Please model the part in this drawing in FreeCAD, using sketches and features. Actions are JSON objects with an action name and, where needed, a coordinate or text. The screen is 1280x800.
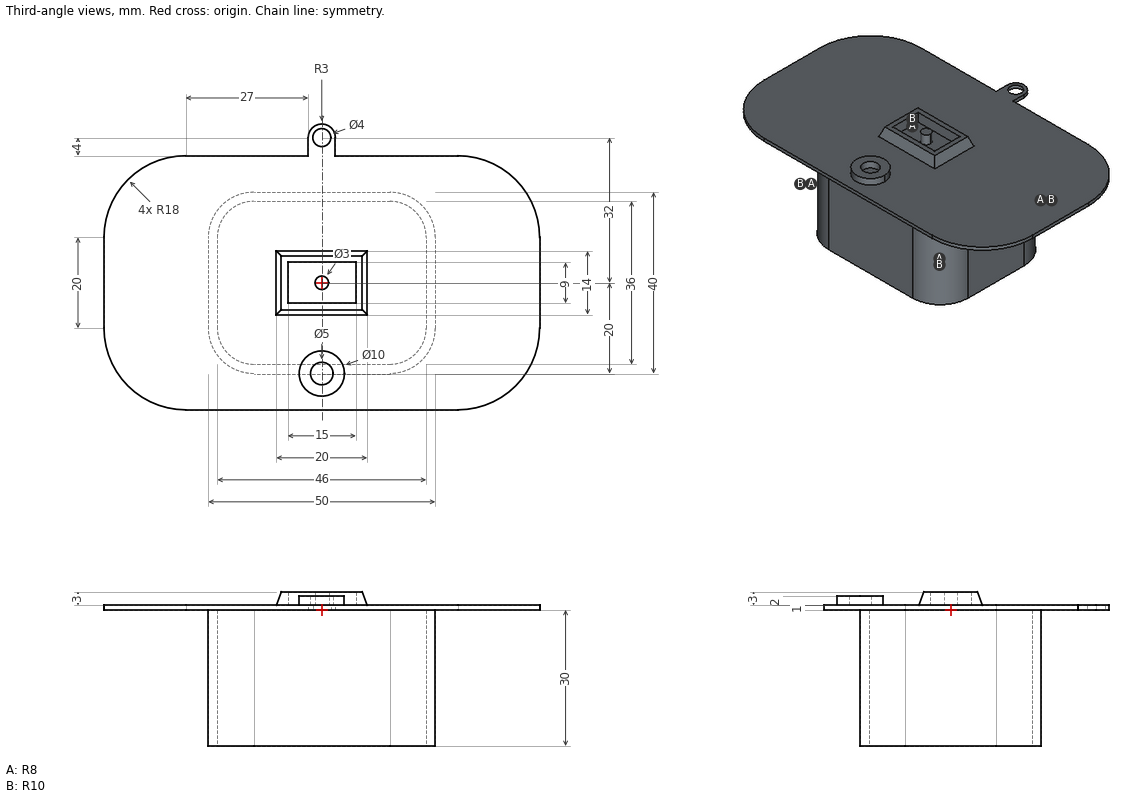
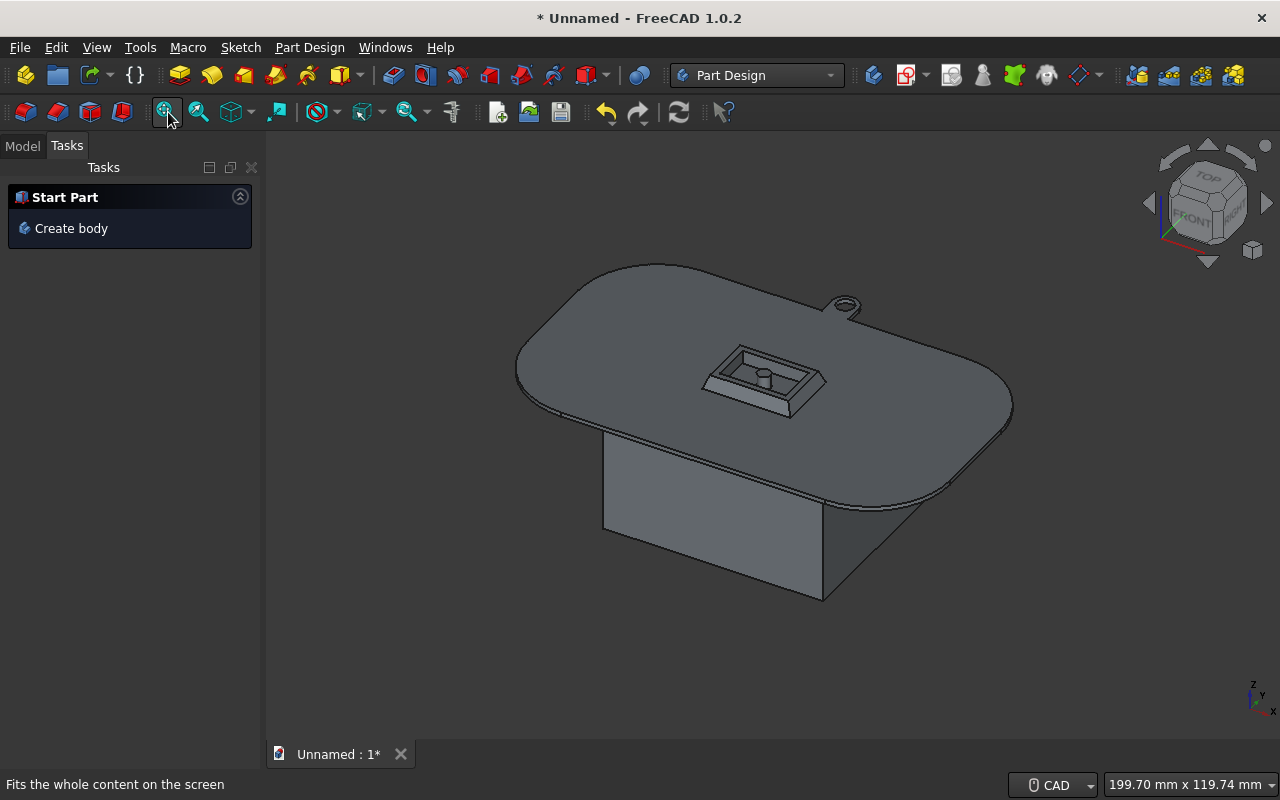
{"action": "left_click", "coordinate": [652, 336]}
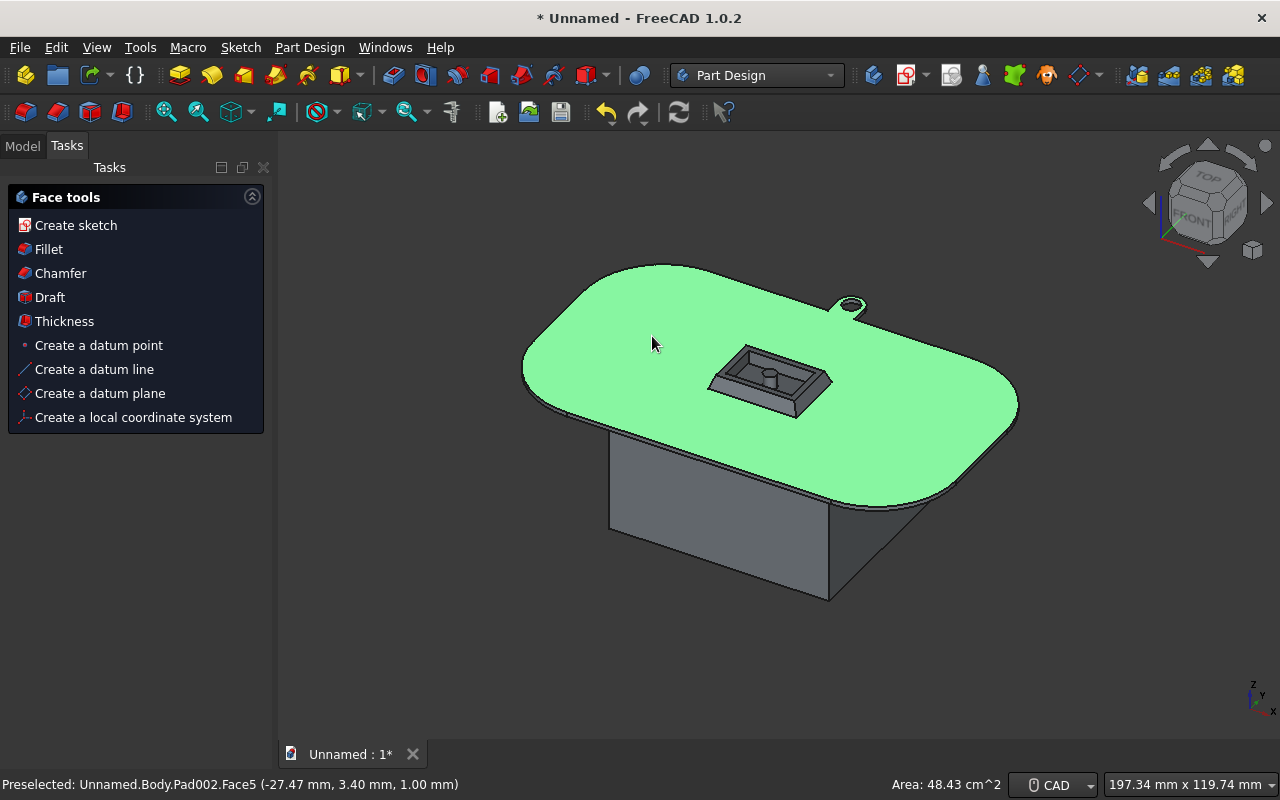
{"action": "left_click", "coordinate": [906, 76]}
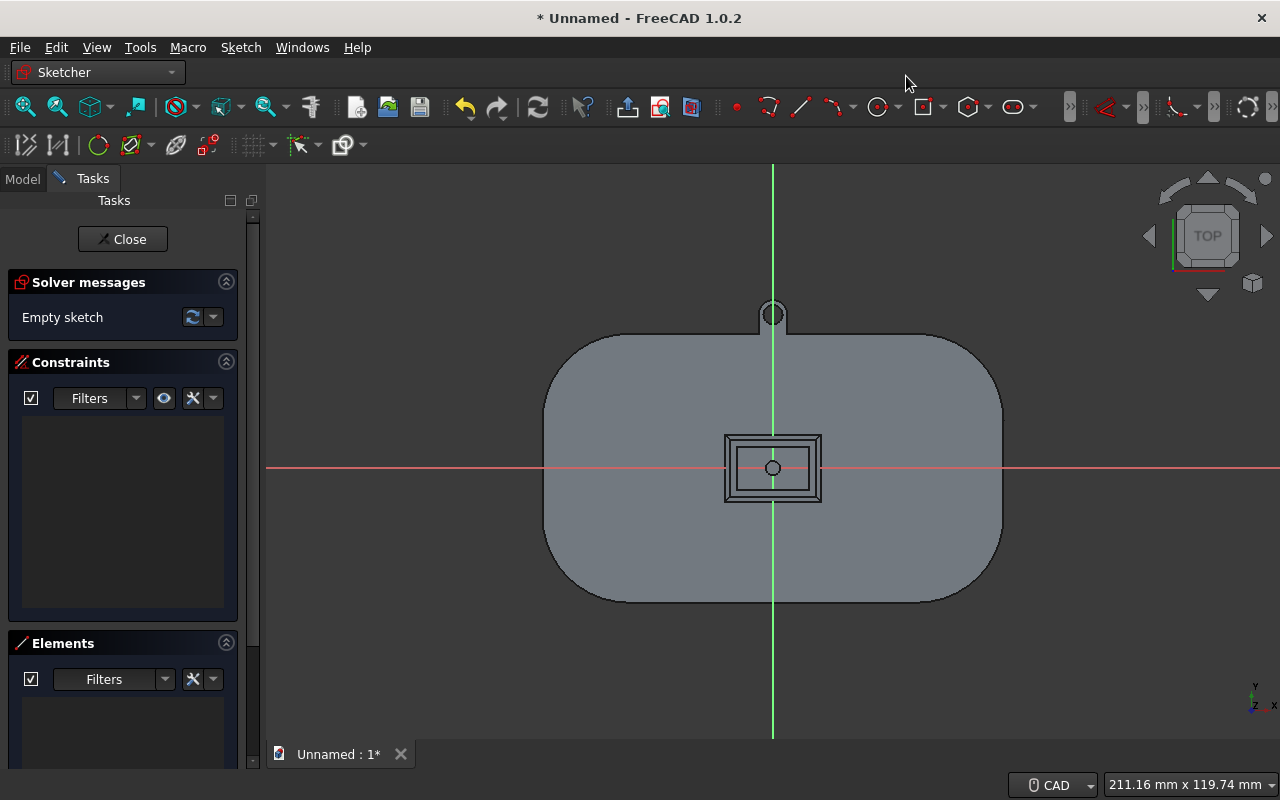
{"action": "left_click", "coordinate": [692, 108]}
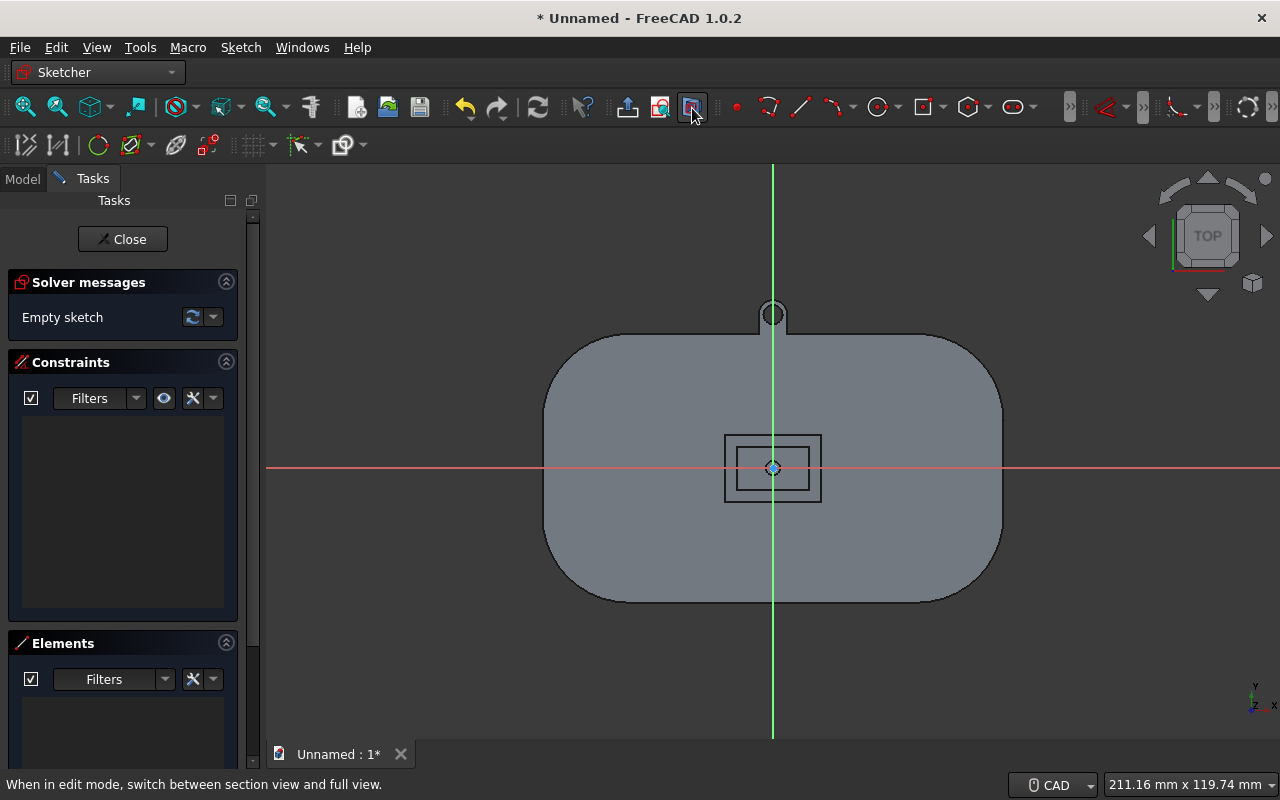
{"action": "scroll", "coordinate": [784, 582], "scroll_direction": "up", "scroll_amount": 10}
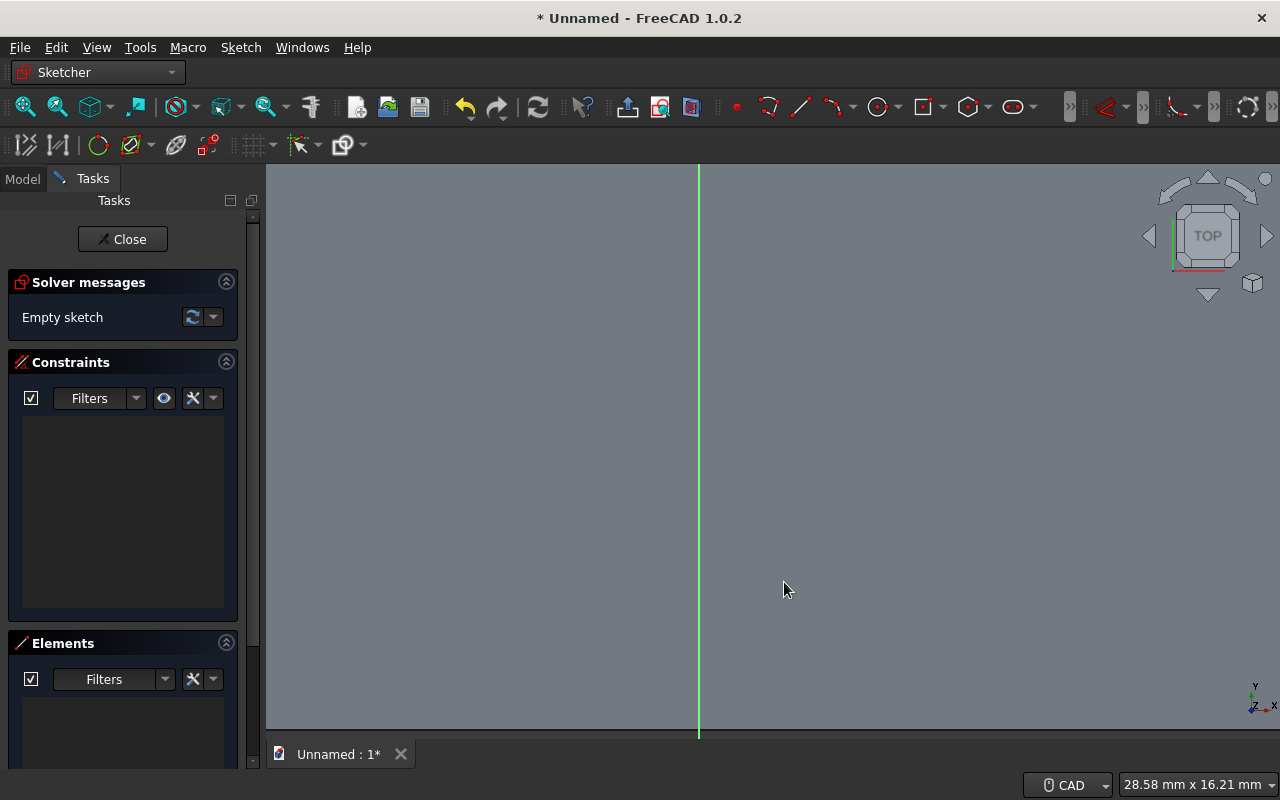
{"action": "left_click", "coordinate": [878, 108]}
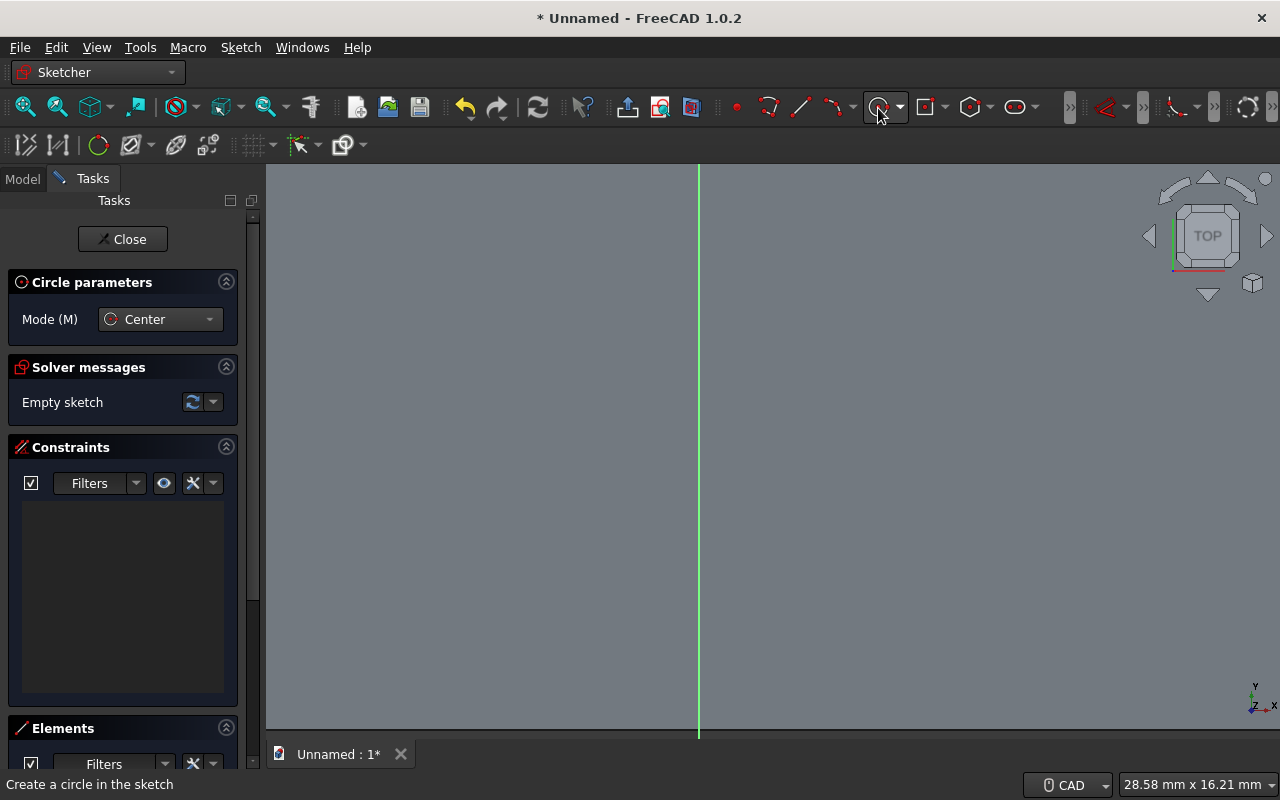
{"action": "left_click", "coordinate": [699, 447]}
{"action": "mouse_move", "coordinate": [825, 321]}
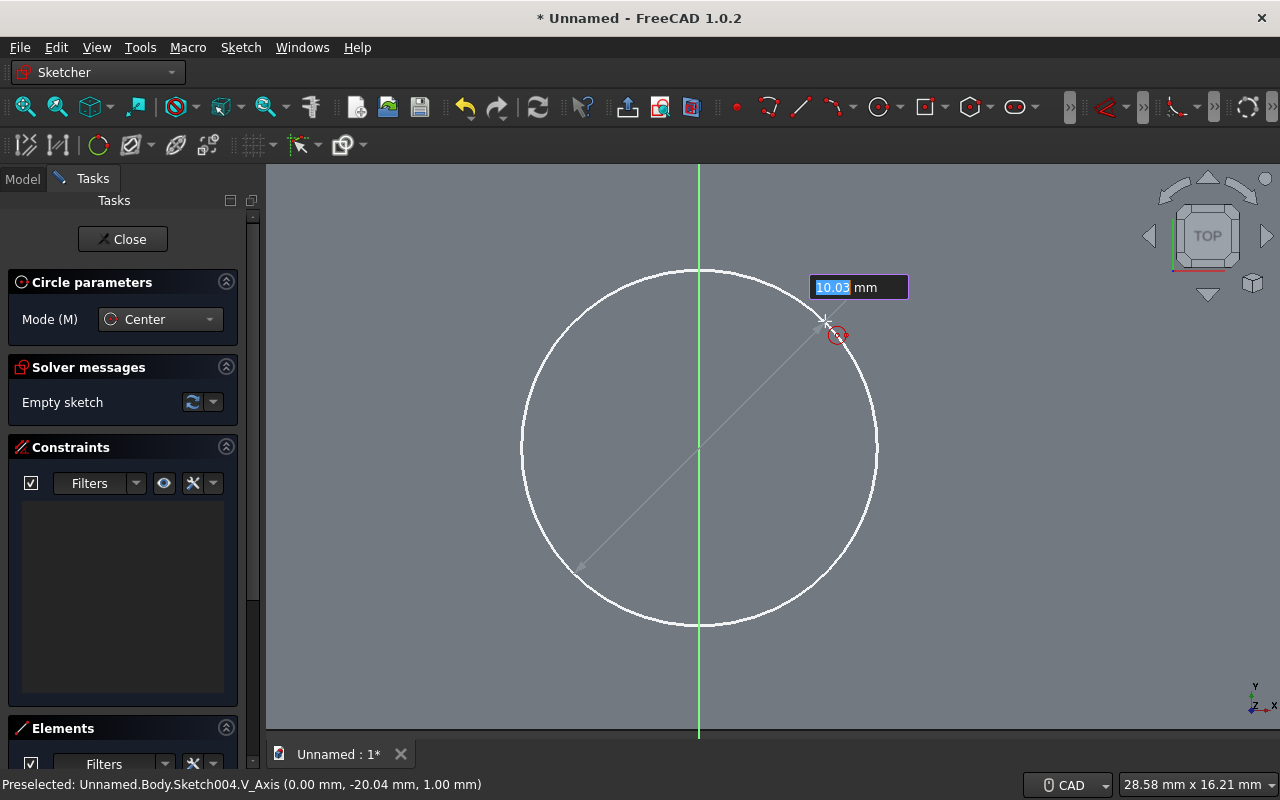
{"action": "type", "text": "10"}
{"action": "key", "text": "Return"}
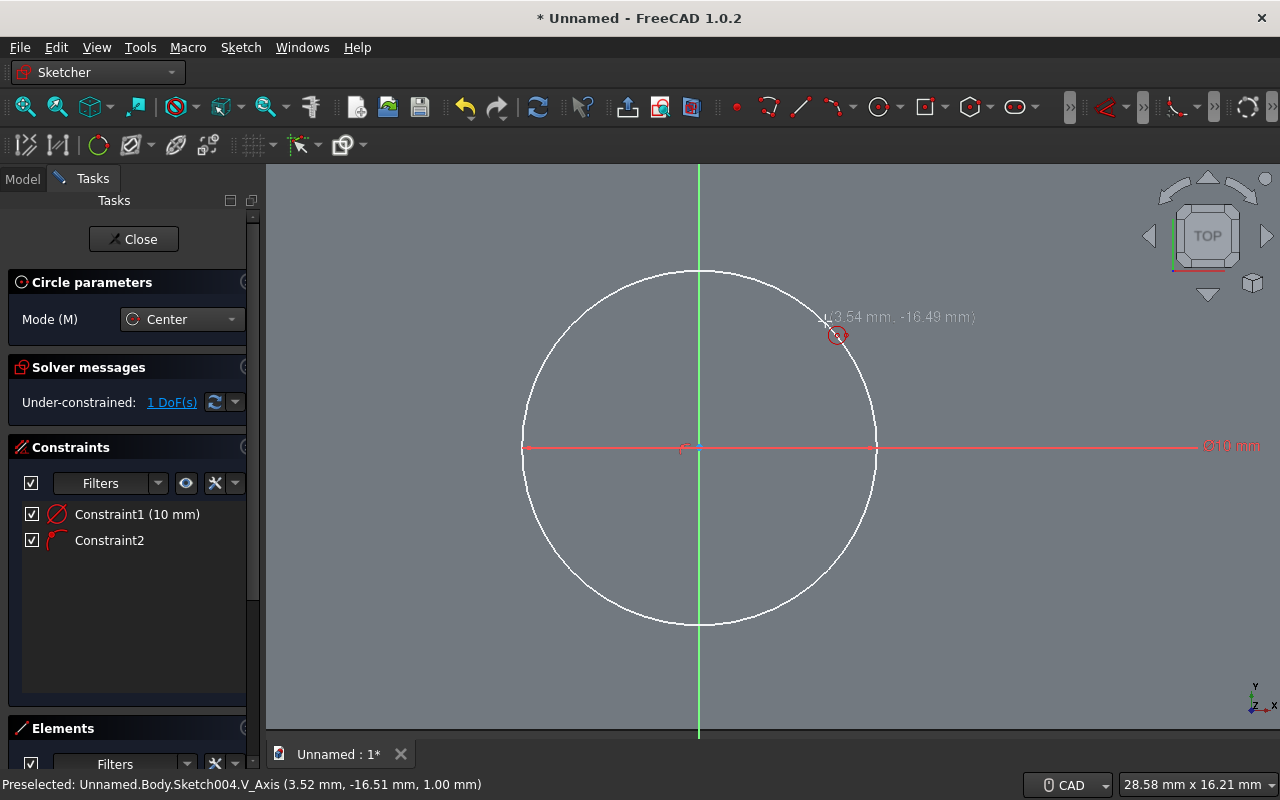
{"action": "left_click", "coordinate": [699, 448]}
{"action": "mouse_move", "coordinate": [762, 384]}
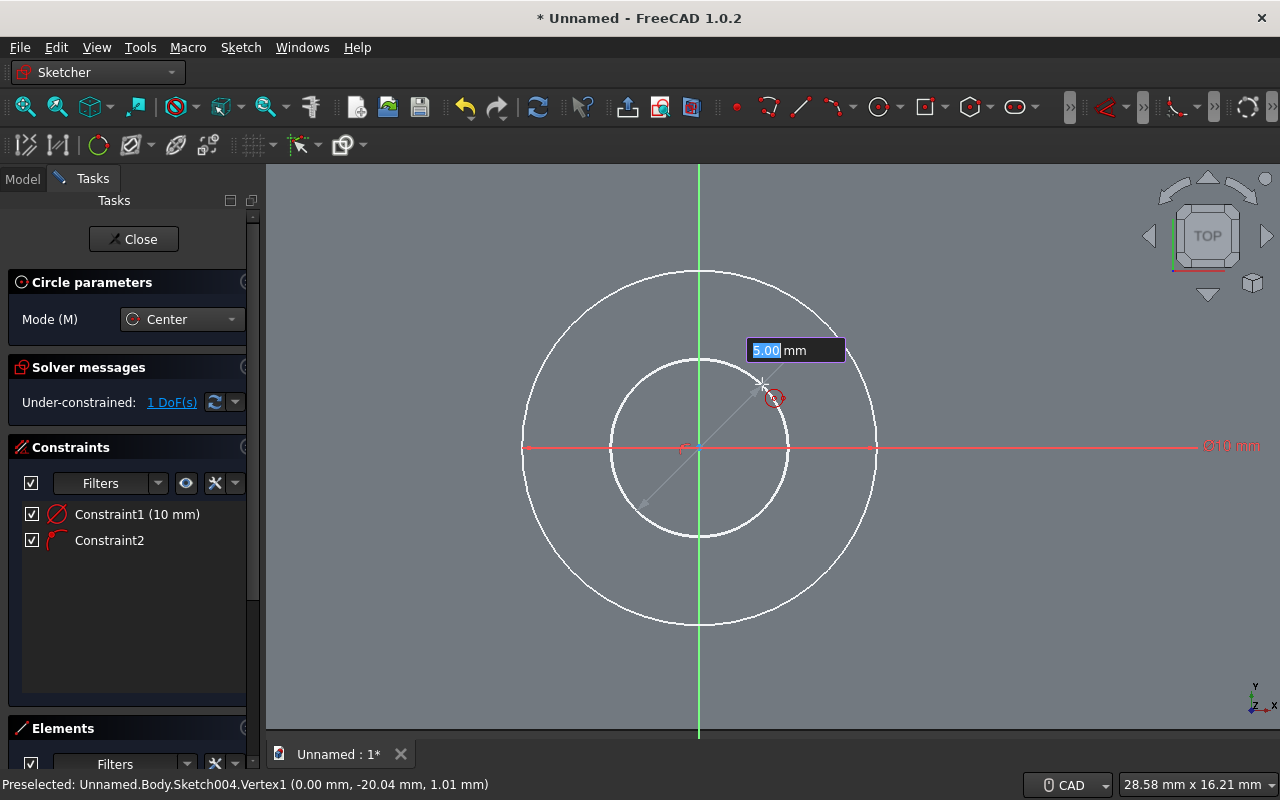
{"action": "type", "text": "5"}
{"action": "key", "text": "Return"}
{"action": "key", "text": "Escape"}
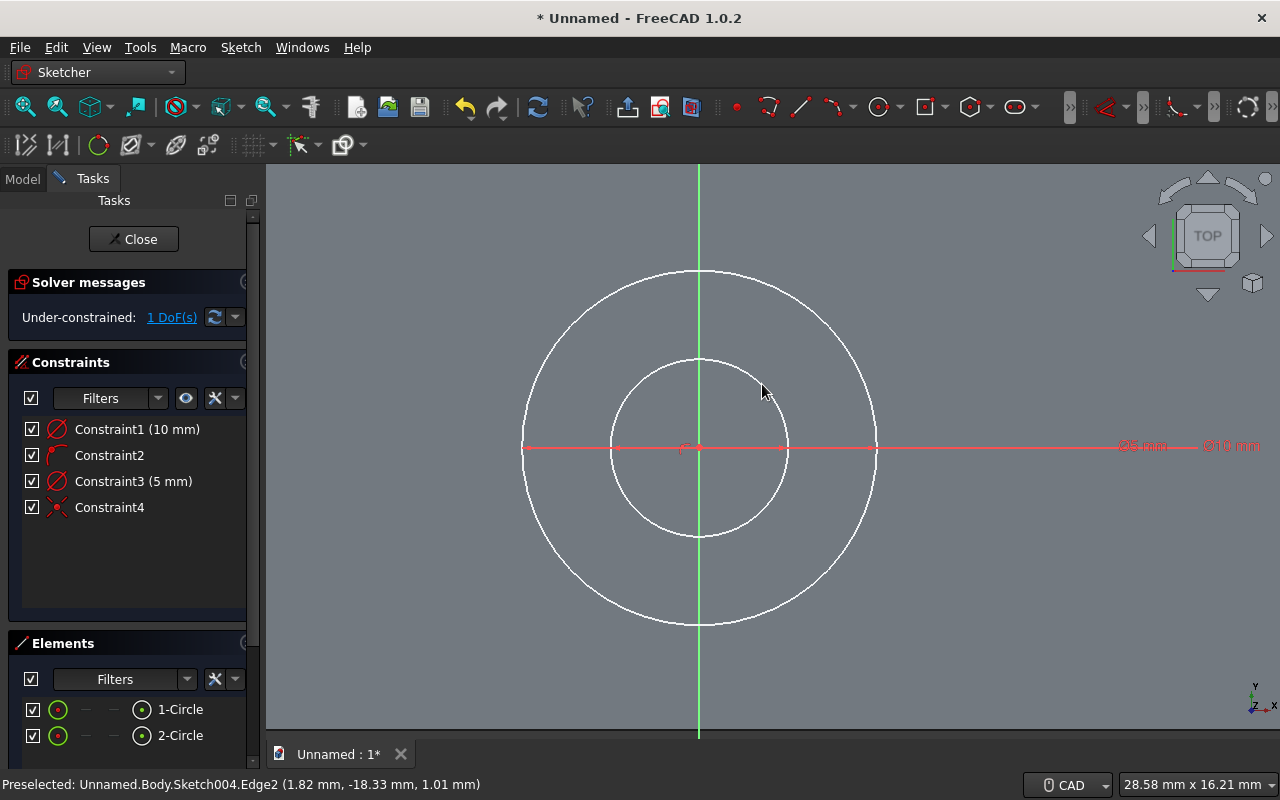
{"action": "left_click", "coordinate": [1106, 108]}